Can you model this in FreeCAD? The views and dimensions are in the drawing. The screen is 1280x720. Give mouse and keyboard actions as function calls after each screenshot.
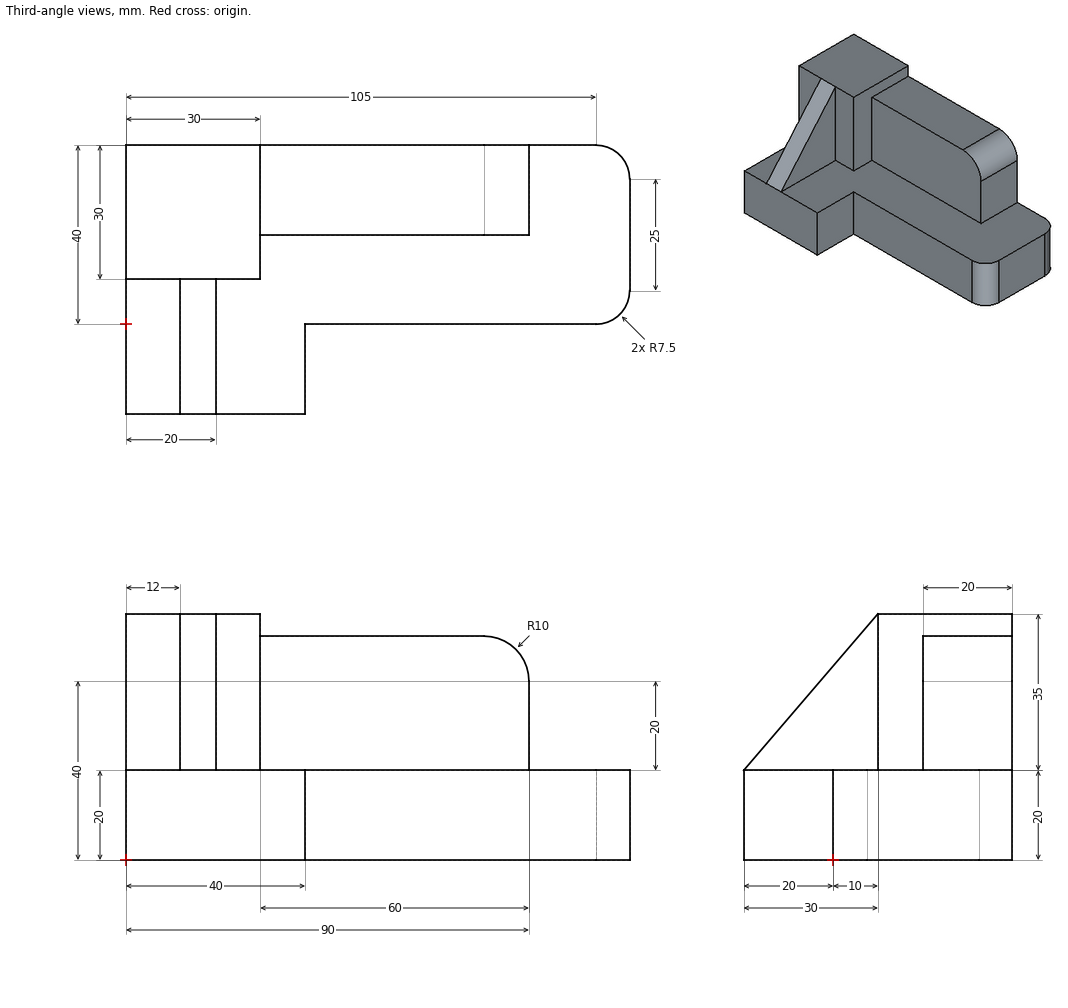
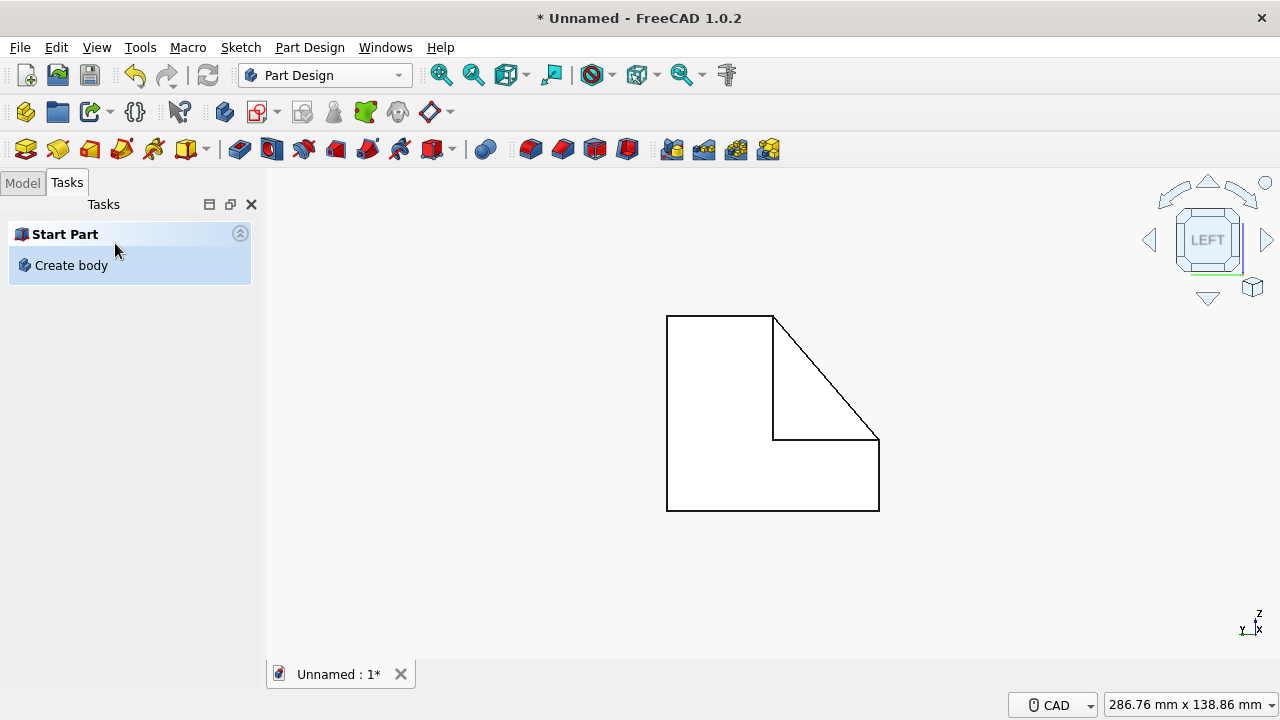
key(0)